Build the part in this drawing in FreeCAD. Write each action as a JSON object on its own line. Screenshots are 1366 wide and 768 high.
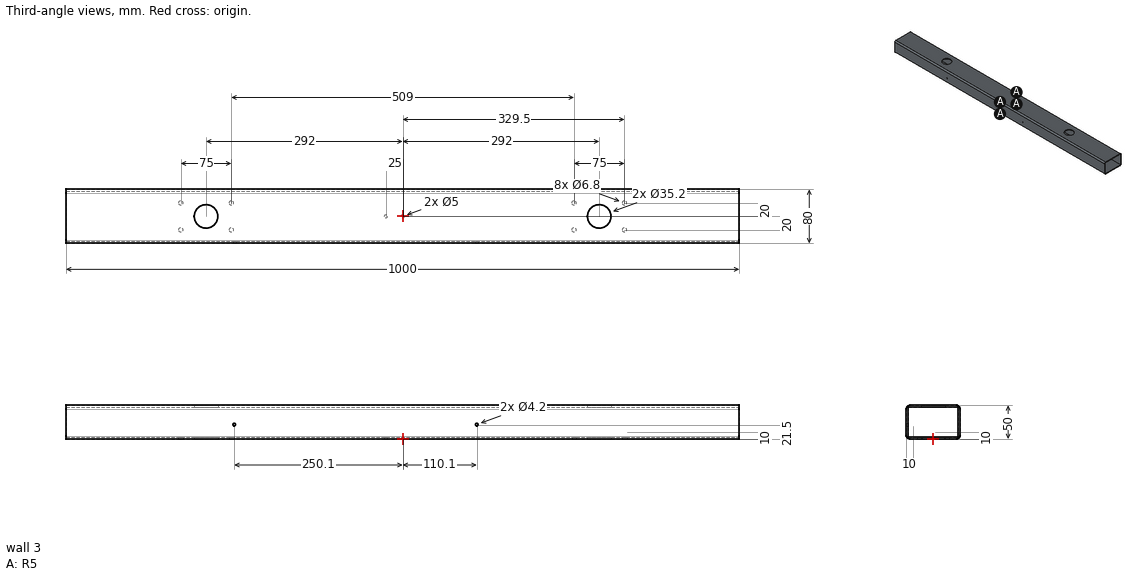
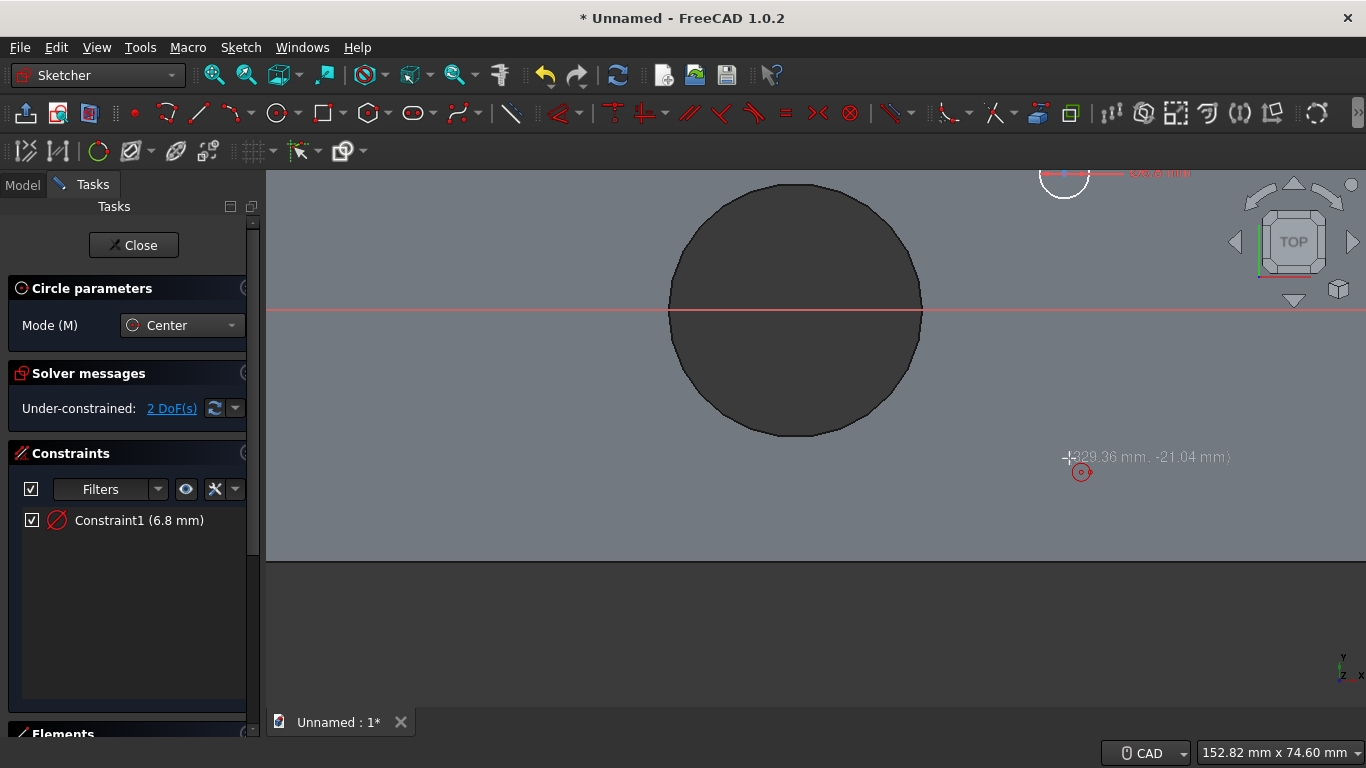
{"action": "scroll", "coordinate": [1069, 459], "scroll_direction": "down", "scroll_amount": 10}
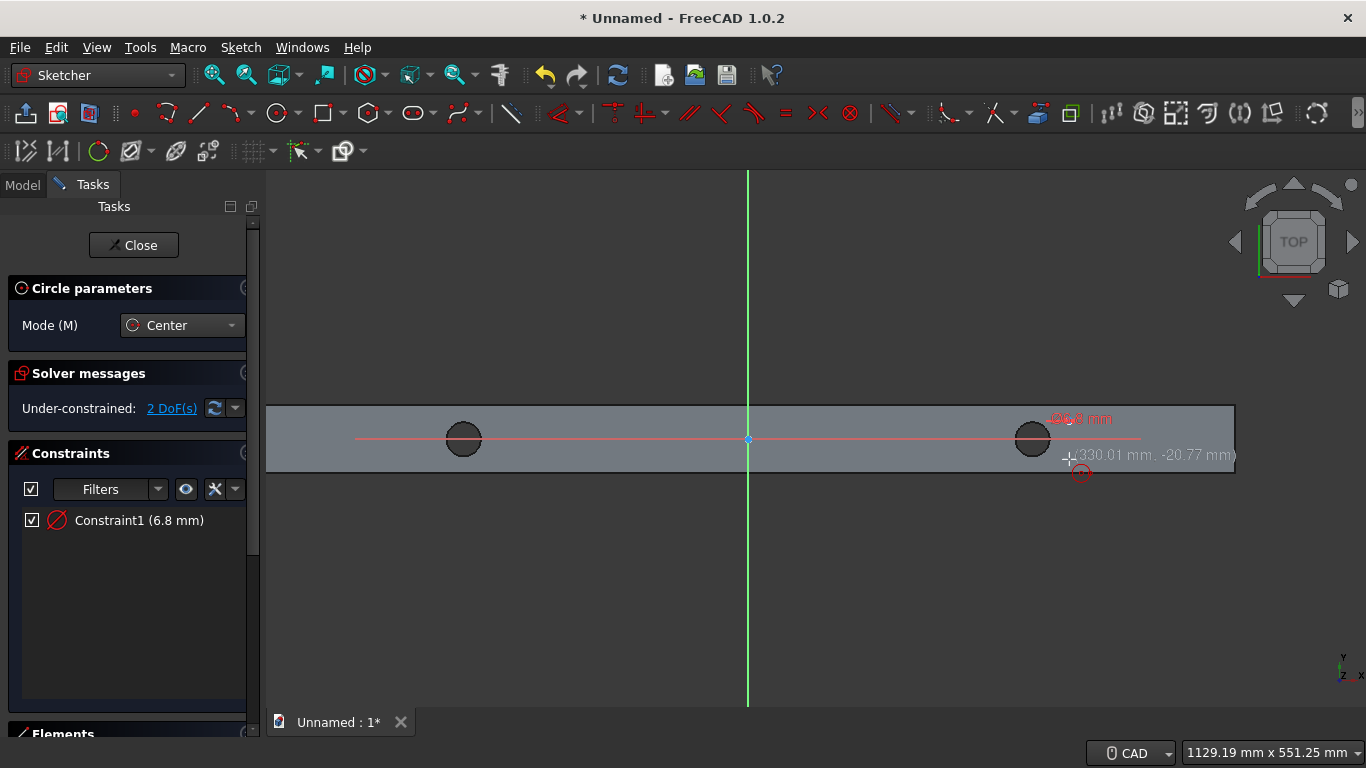
{"action": "left_click", "coordinate": [1069, 459]}
{"action": "mouse_move", "coordinate": [1071, 457]}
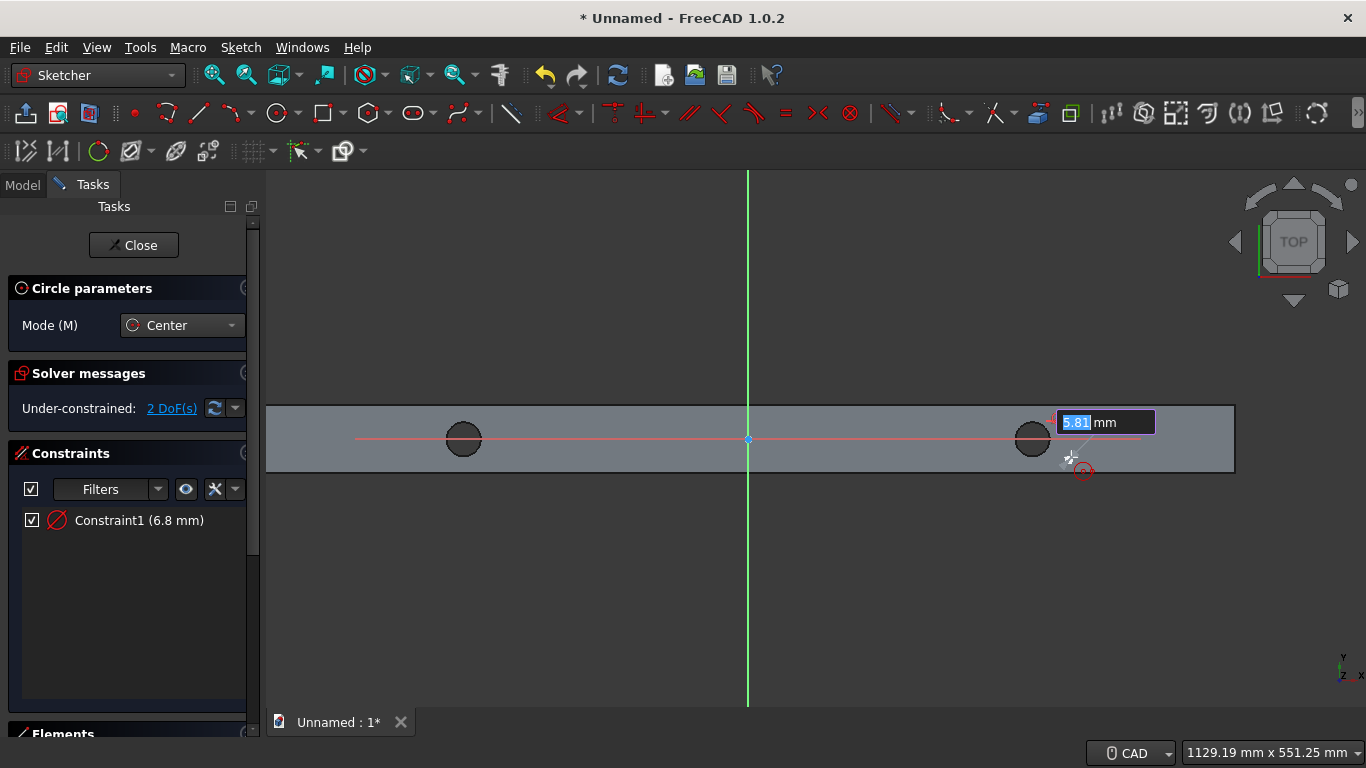
{"action": "type", "text": "6.8"}
{"action": "key", "text": "Return"}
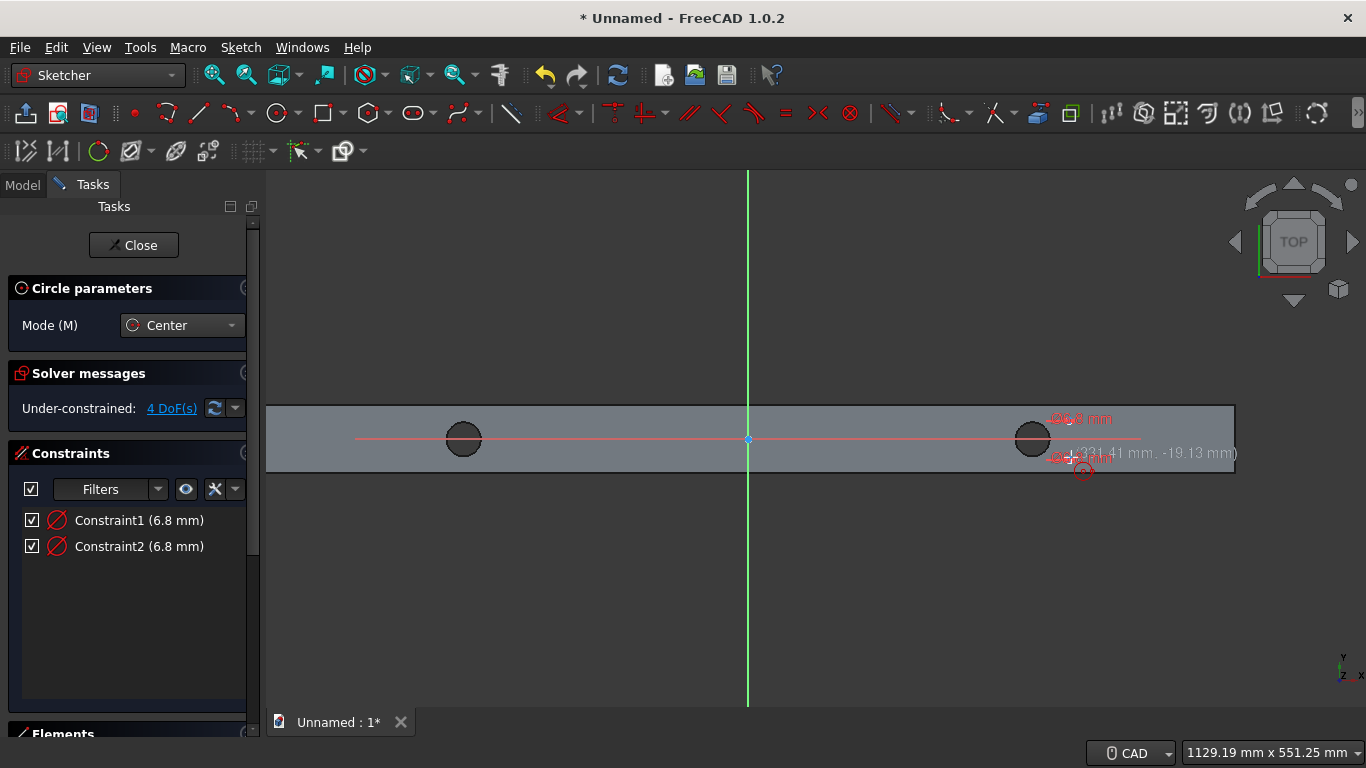
{"action": "scroll", "coordinate": [996, 420], "scroll_direction": "up", "scroll_amount": 10}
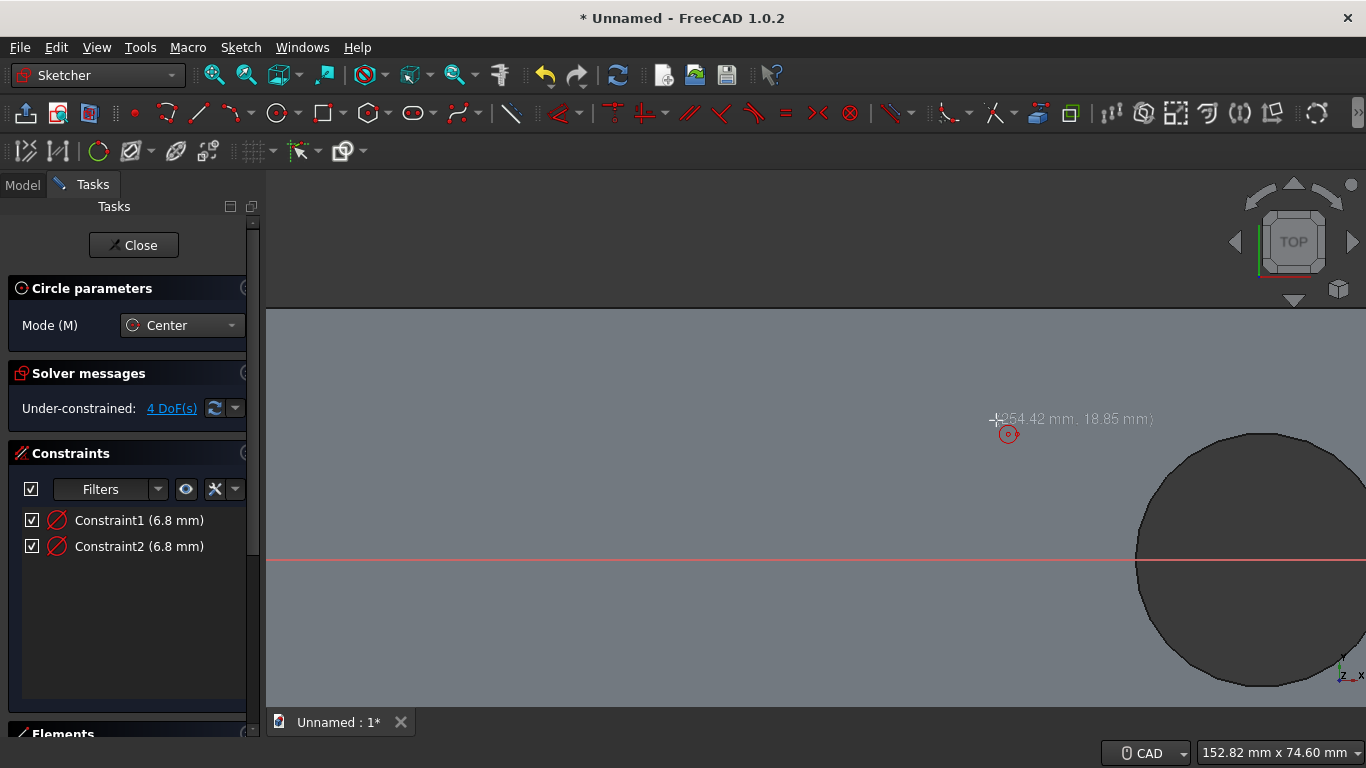
{"action": "scroll", "coordinate": [996, 419], "scroll_direction": "down", "scroll_amount": 10}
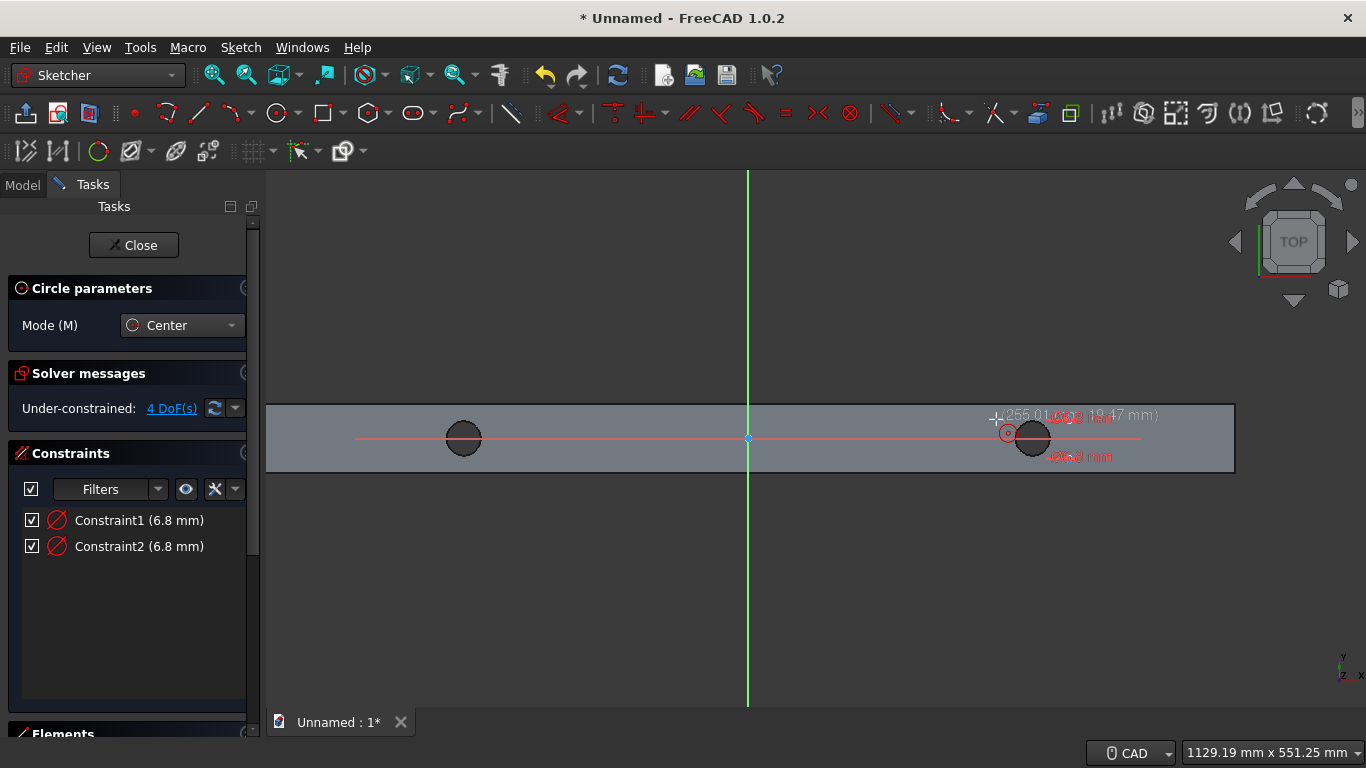
{"action": "left_click", "coordinate": [996, 419]}
{"action": "mouse_move", "coordinate": [998, 417]}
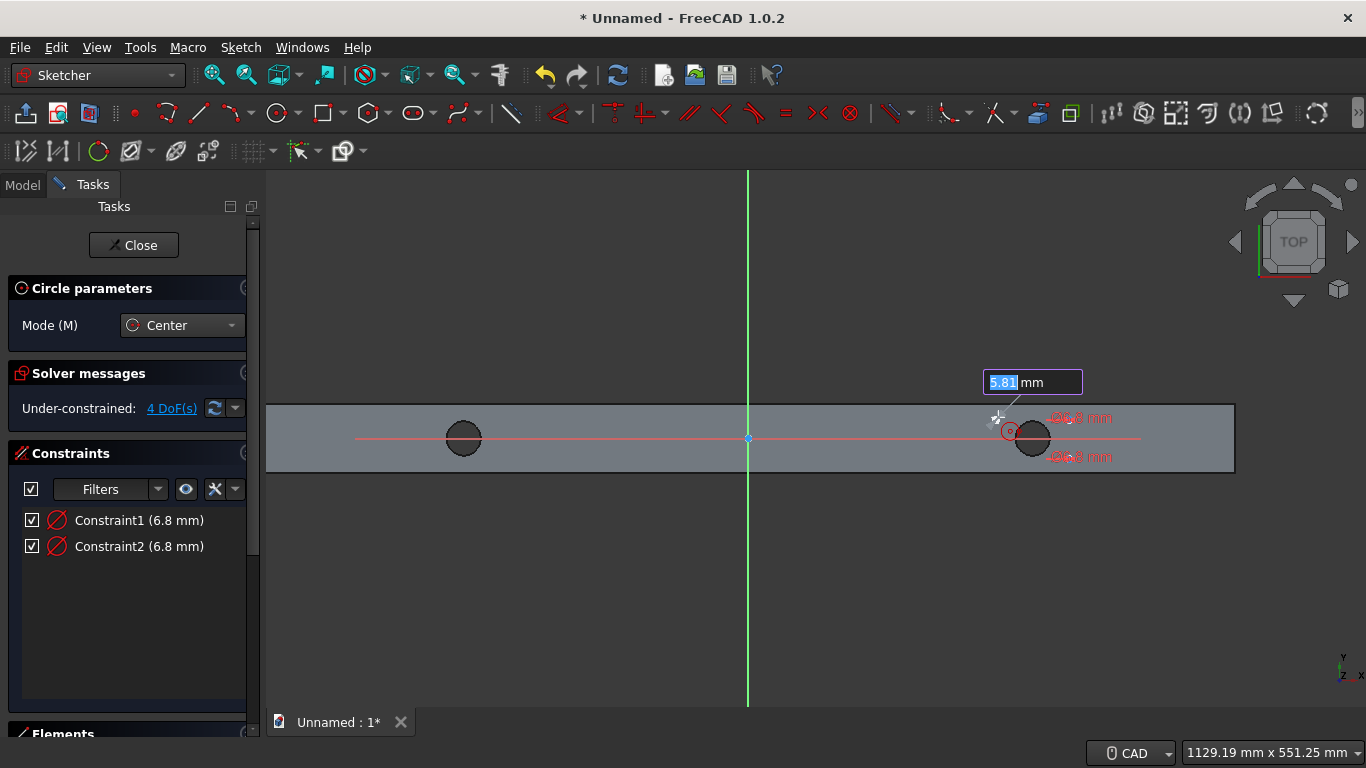
{"action": "type", "text": "6.8"}
{"action": "key", "text": "Return"}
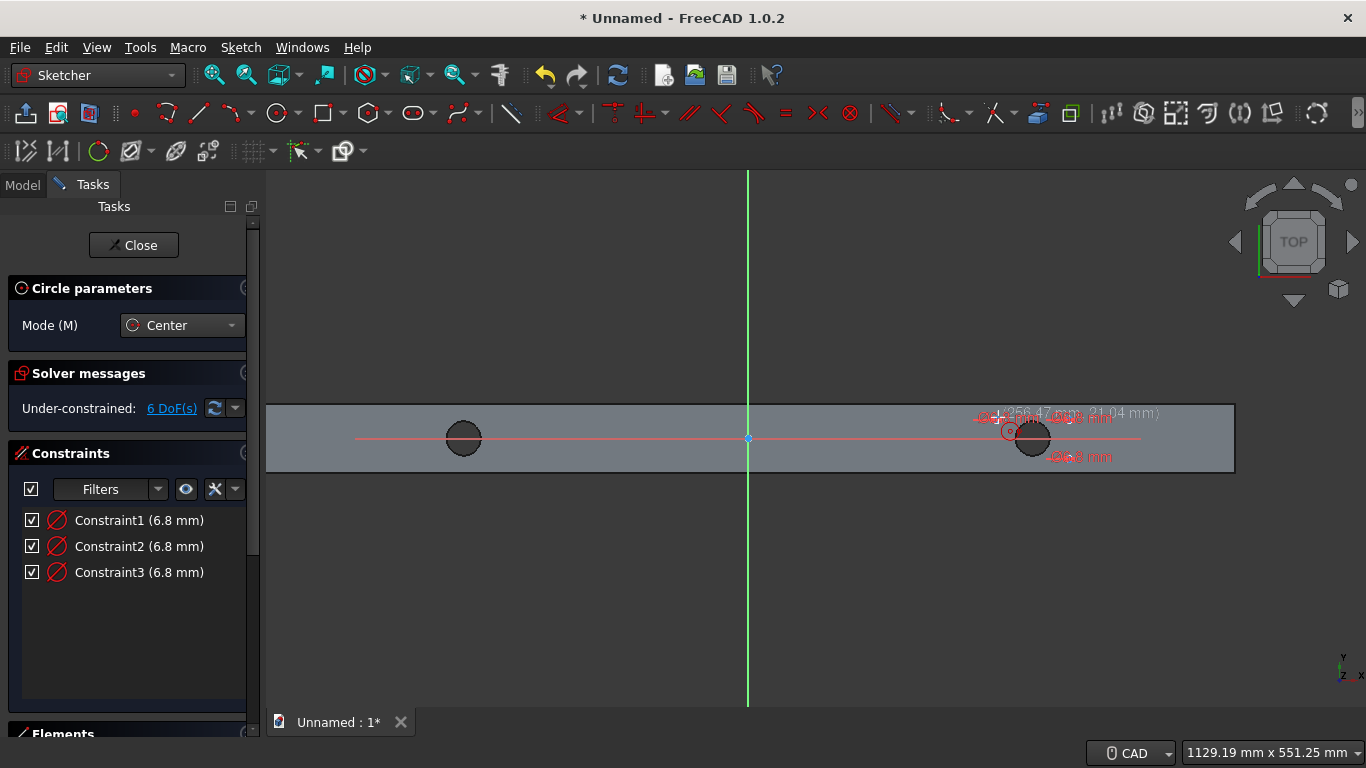
{"action": "scroll", "coordinate": [996, 458], "scroll_direction": "up", "scroll_amount": 10}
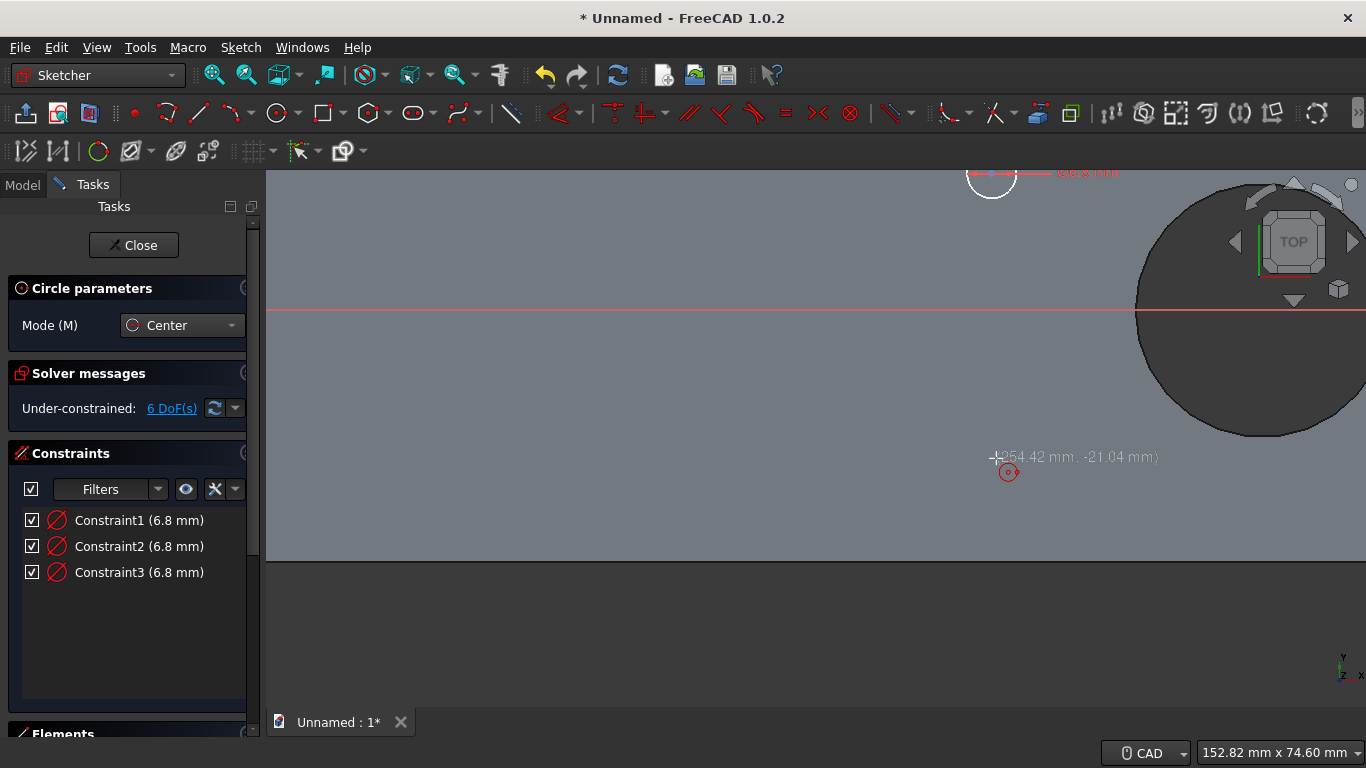
{"action": "scroll", "coordinate": [996, 459], "scroll_direction": "down", "scroll_amount": 10}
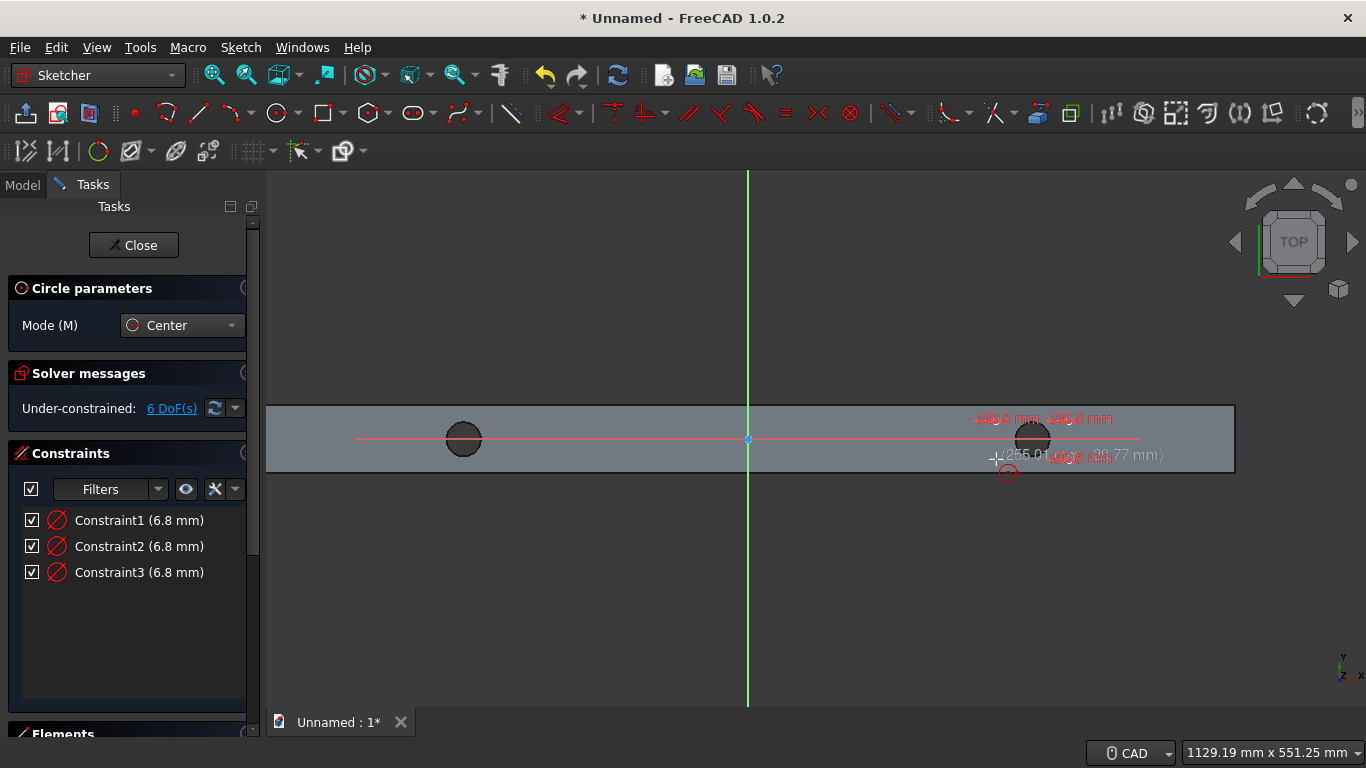
{"action": "left_click", "coordinate": [996, 459]}
{"action": "mouse_move", "coordinate": [998, 457]}